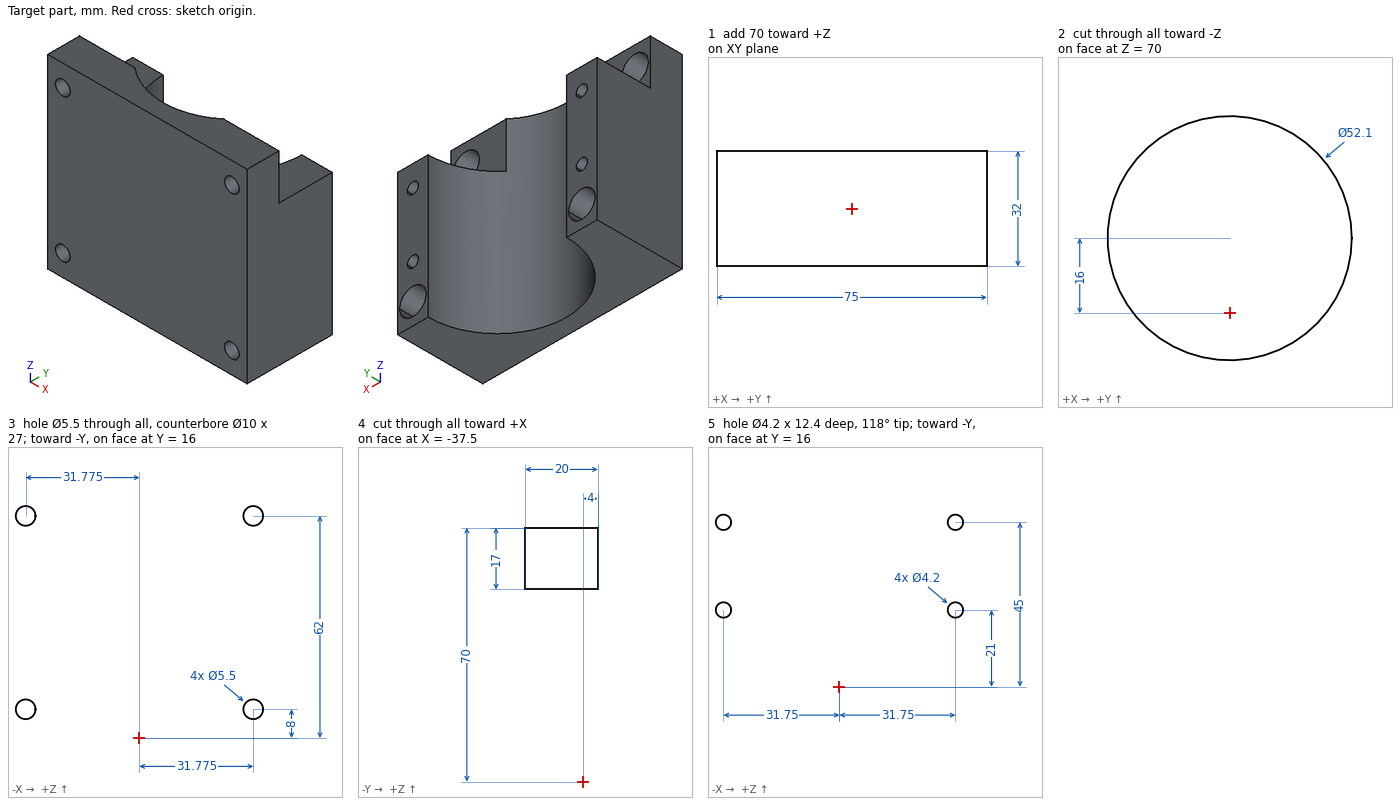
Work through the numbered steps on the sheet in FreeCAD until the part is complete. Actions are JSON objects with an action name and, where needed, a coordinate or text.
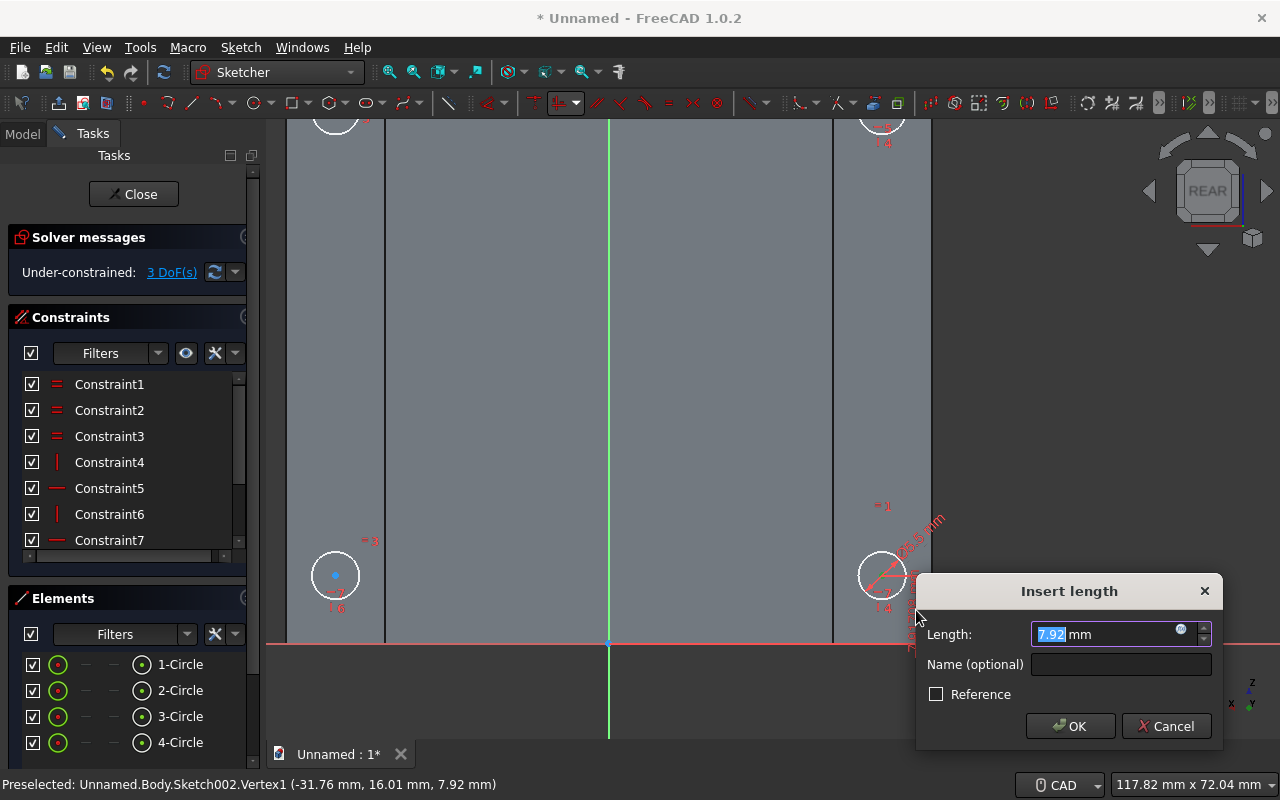
{"action": "type", "text": "8"}
{"action": "key", "text": "Return"}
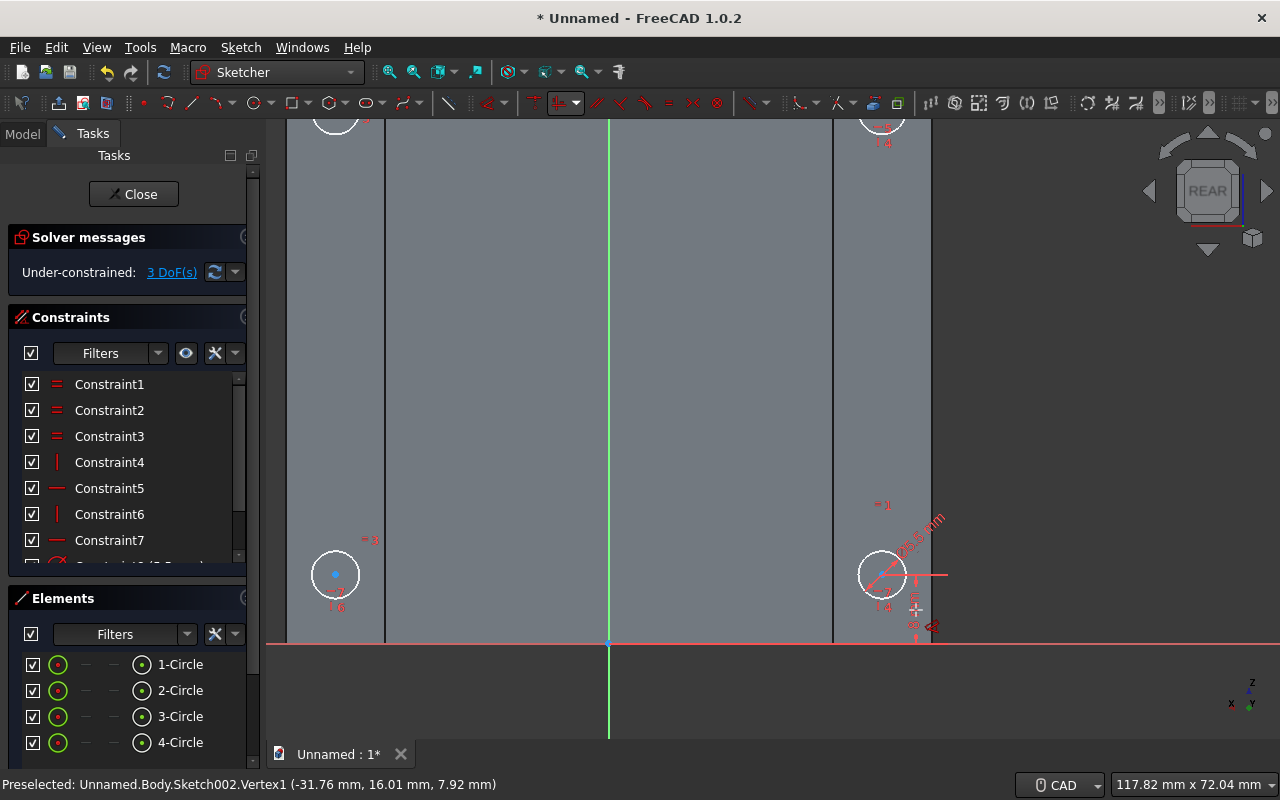
{"action": "scroll", "coordinate": [899, 559], "scroll_direction": "down", "scroll_amount": 2}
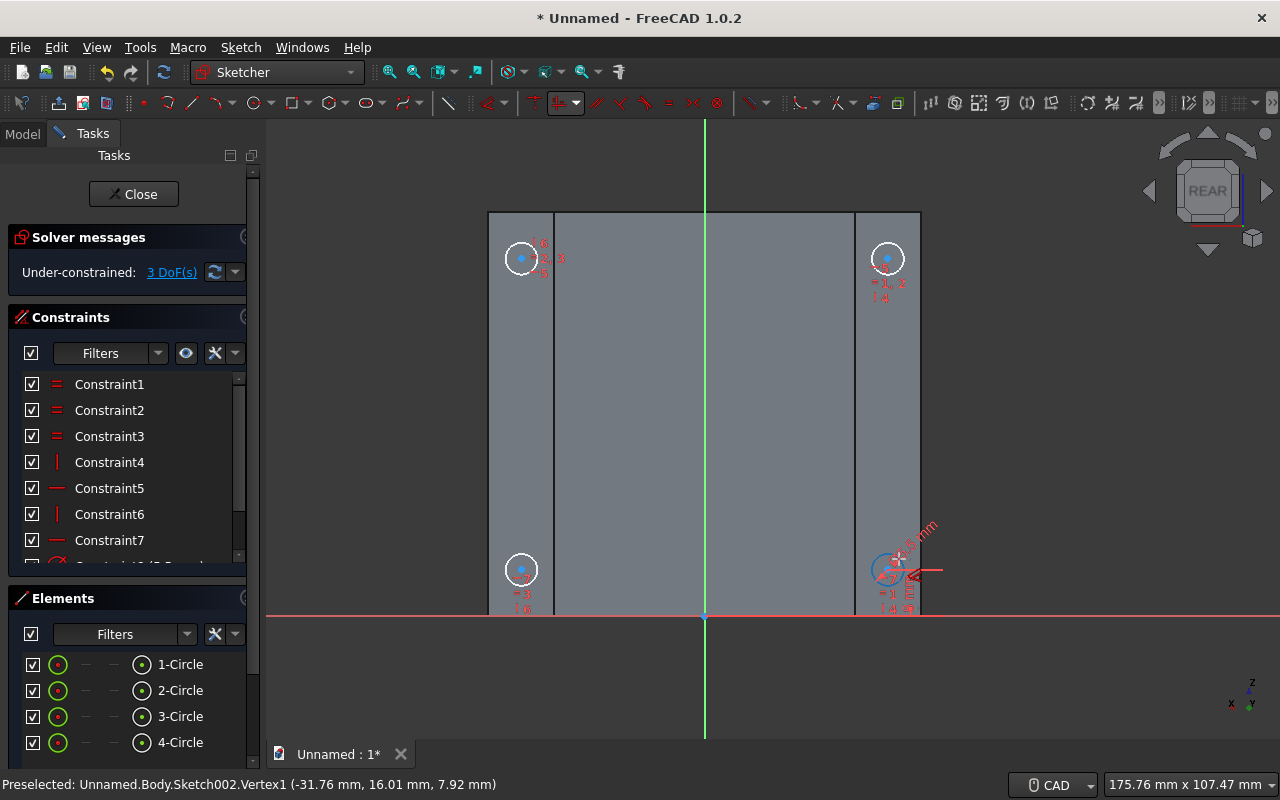
{"action": "left_click", "coordinate": [888, 259]}
{"action": "left_click", "coordinate": [922, 437]}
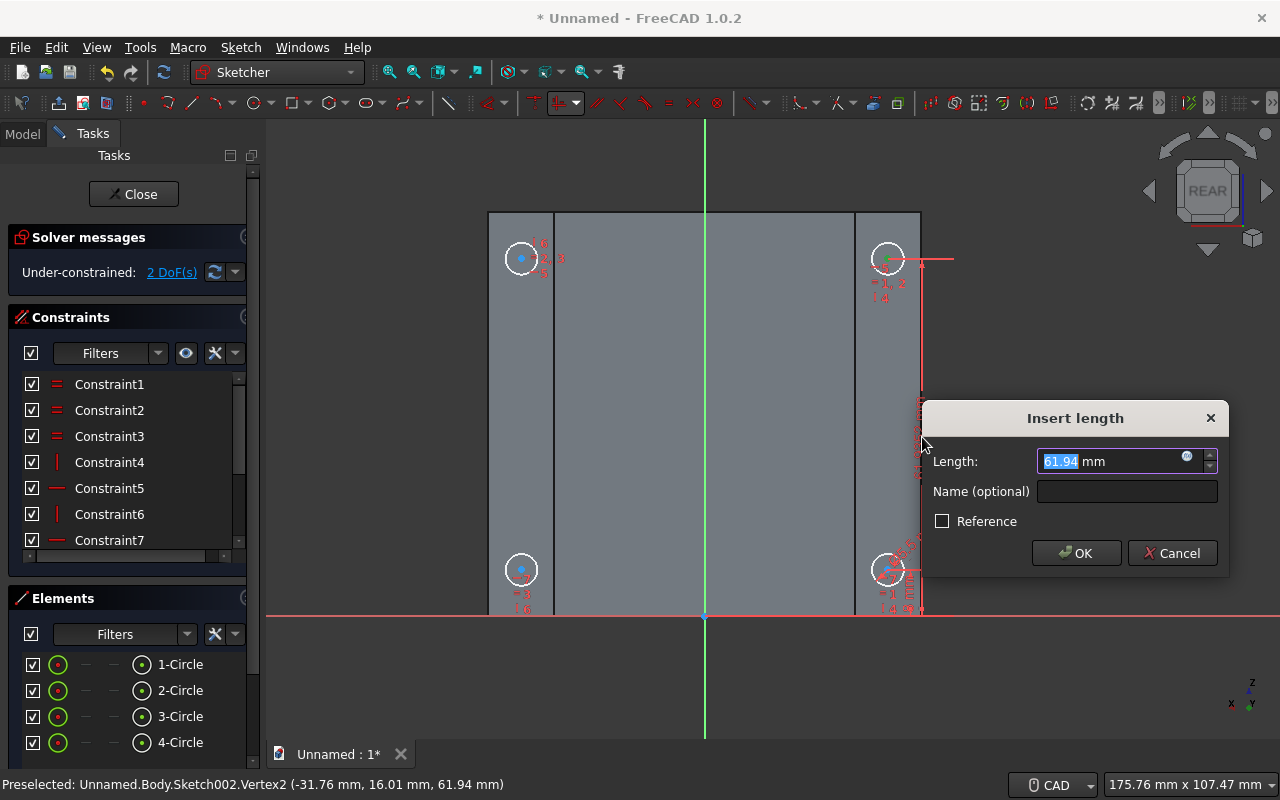
{"action": "type", "text": "62"}
{"action": "key", "text": "Return"}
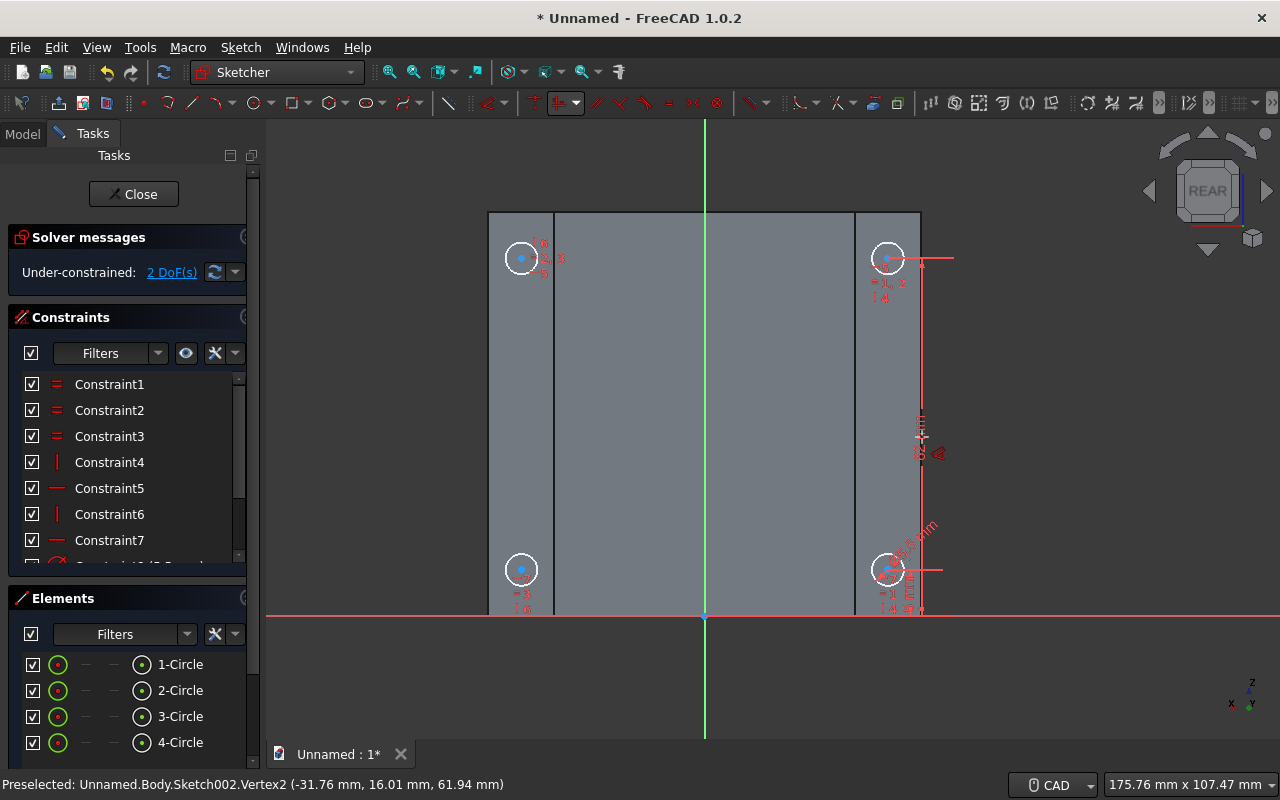
{"action": "left_click", "coordinate": [888, 570]}
{"action": "left_click", "coordinate": [796, 650]}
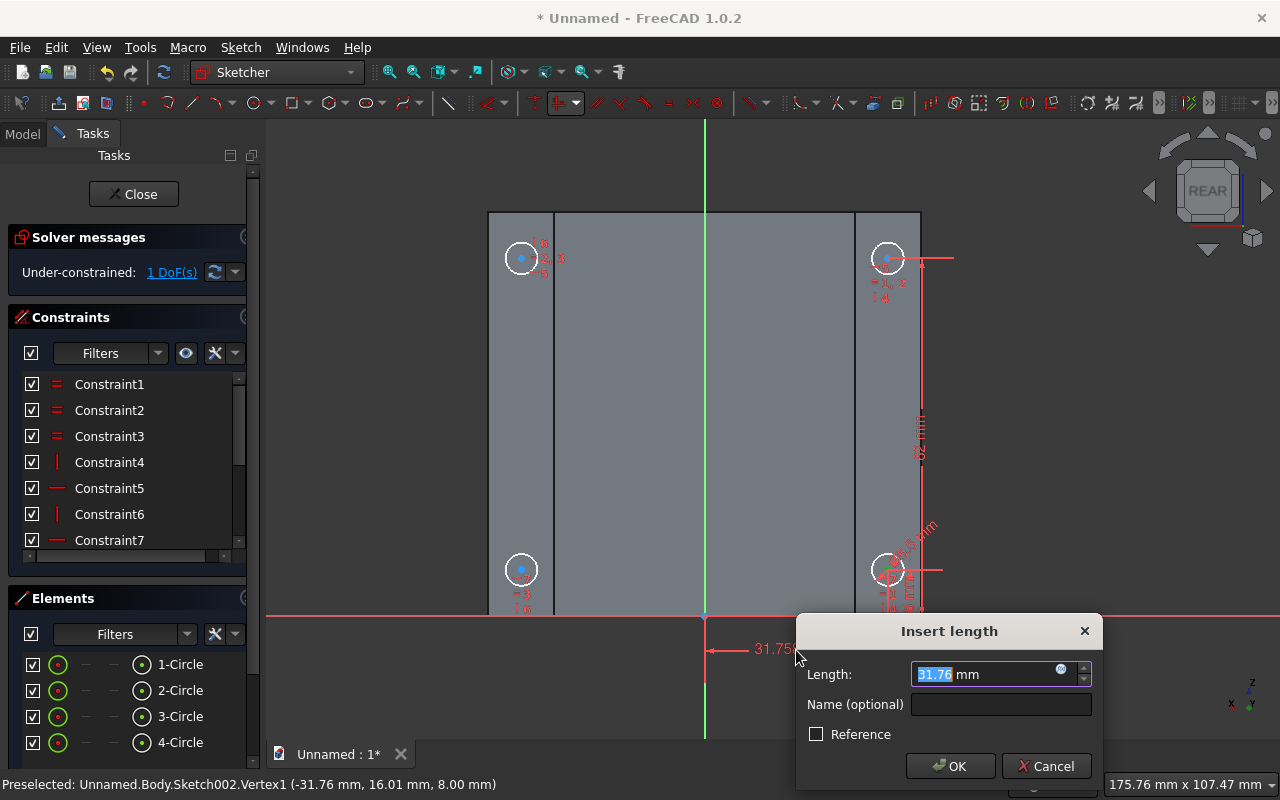
{"action": "type", "text": "31.775"}
{"action": "key", "text": "Return"}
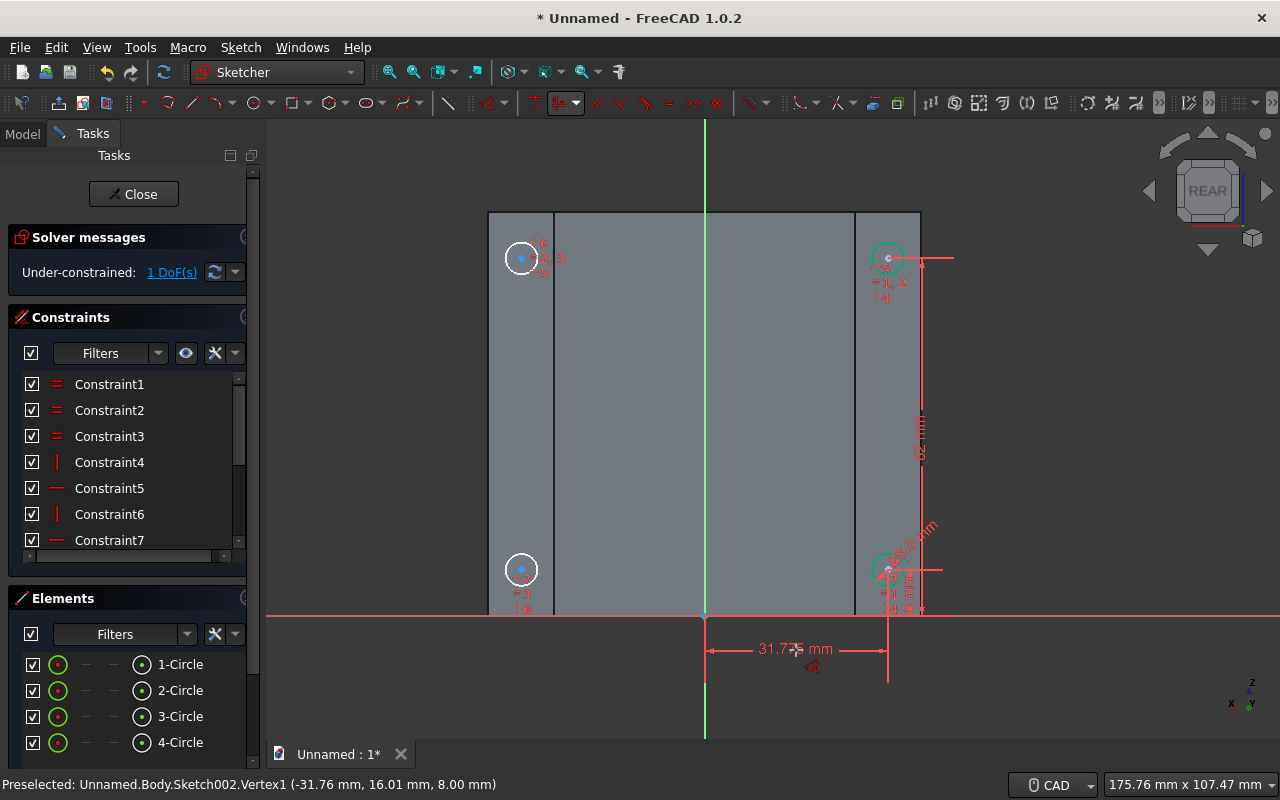
{"action": "left_click", "coordinate": [522, 258]}
{"action": "left_click", "coordinate": [613, 650]}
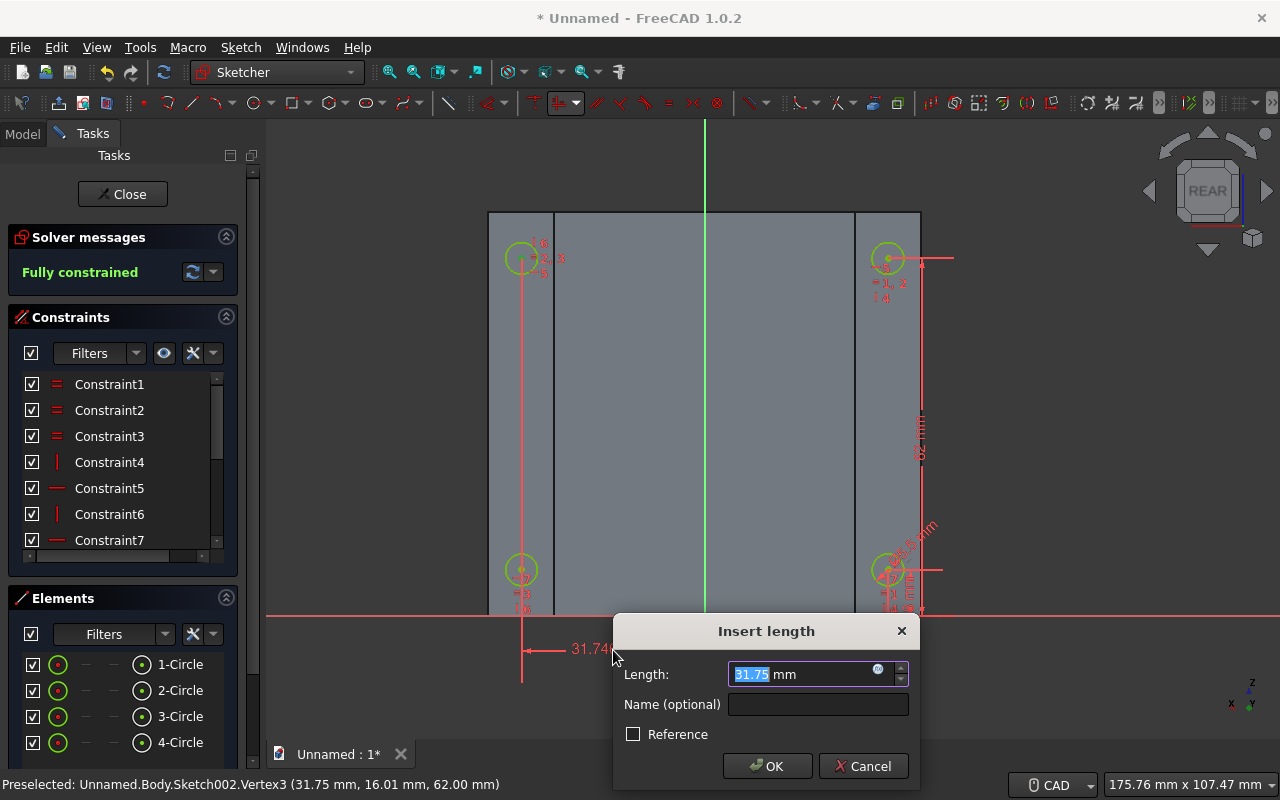
{"action": "type", "text": "31.775"}
{"action": "key", "text": "Return"}
{"action": "key", "text": "Escape"}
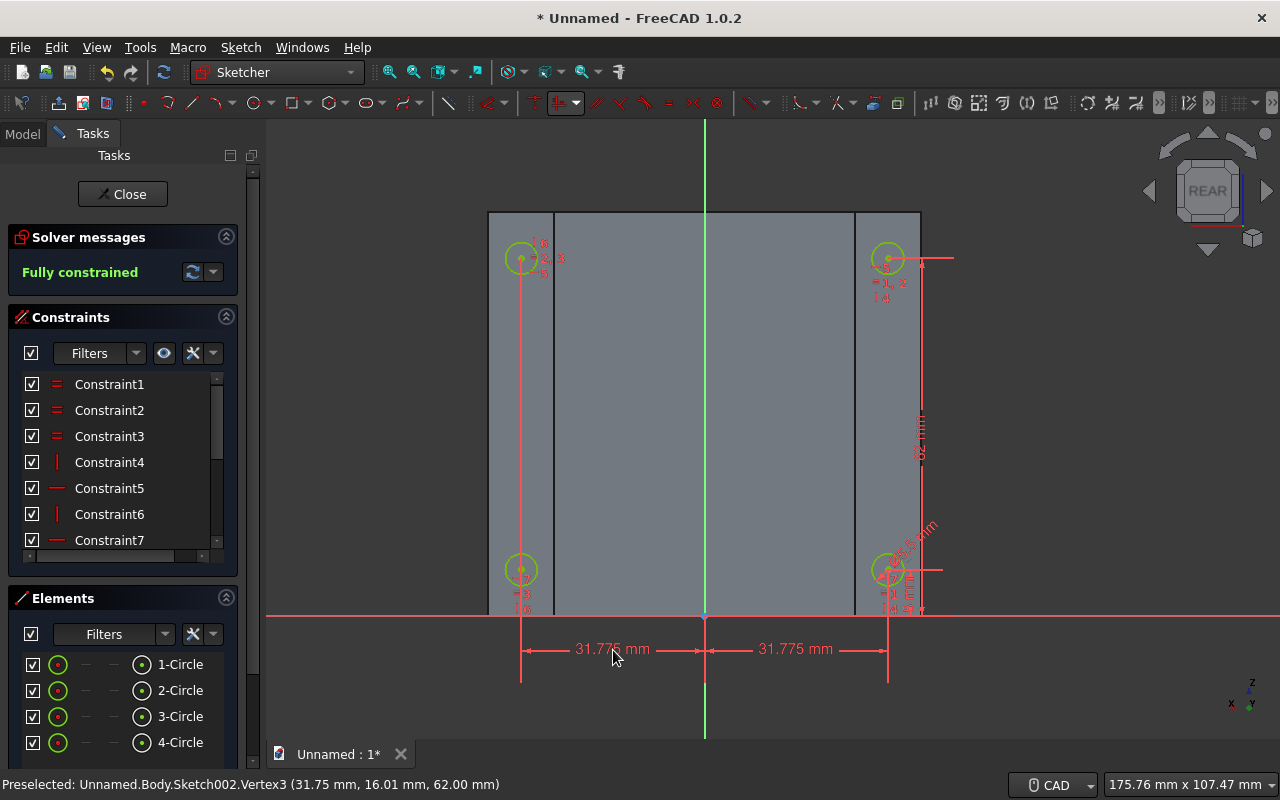
{"action": "left_click", "coordinate": [123, 194]}